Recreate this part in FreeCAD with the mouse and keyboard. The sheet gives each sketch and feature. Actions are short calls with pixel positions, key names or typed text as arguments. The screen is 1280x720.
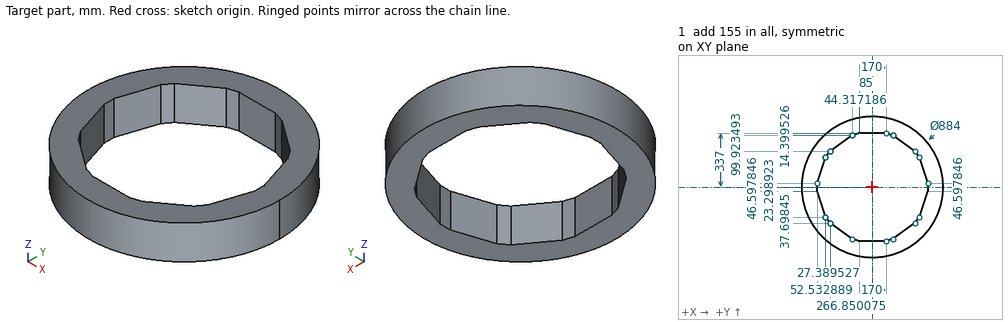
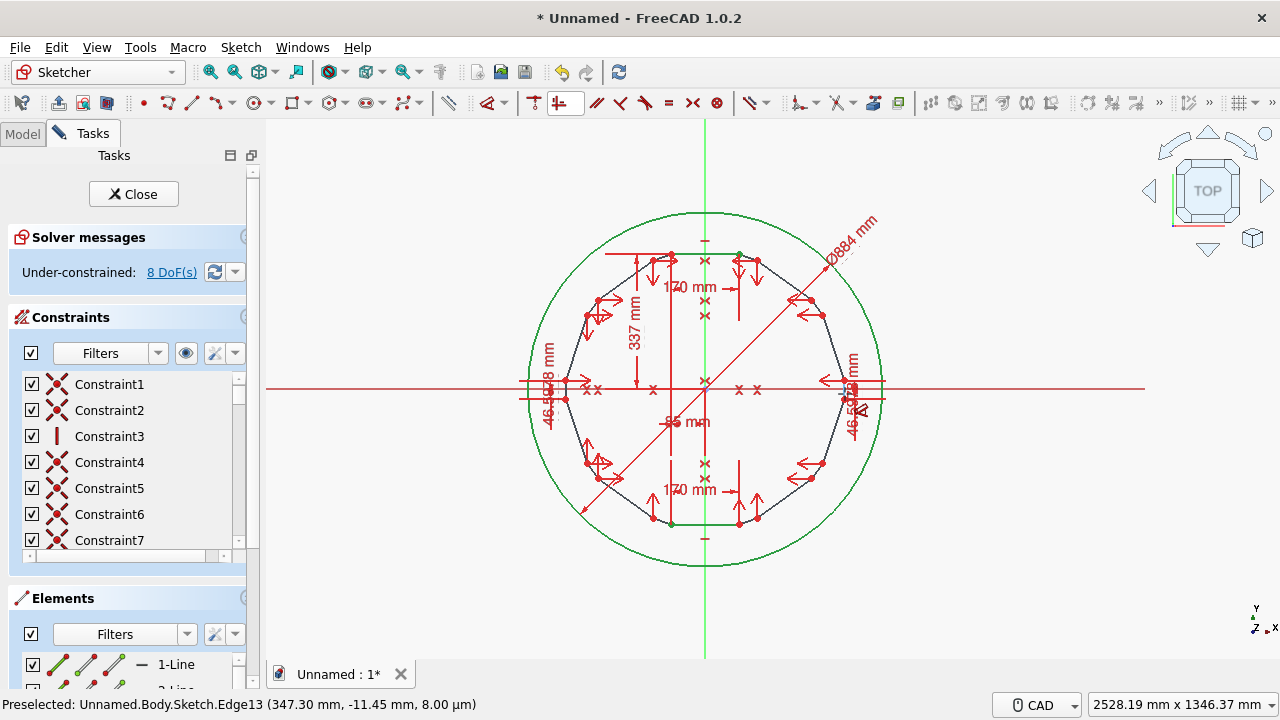
scroll(595, 474, up, 5)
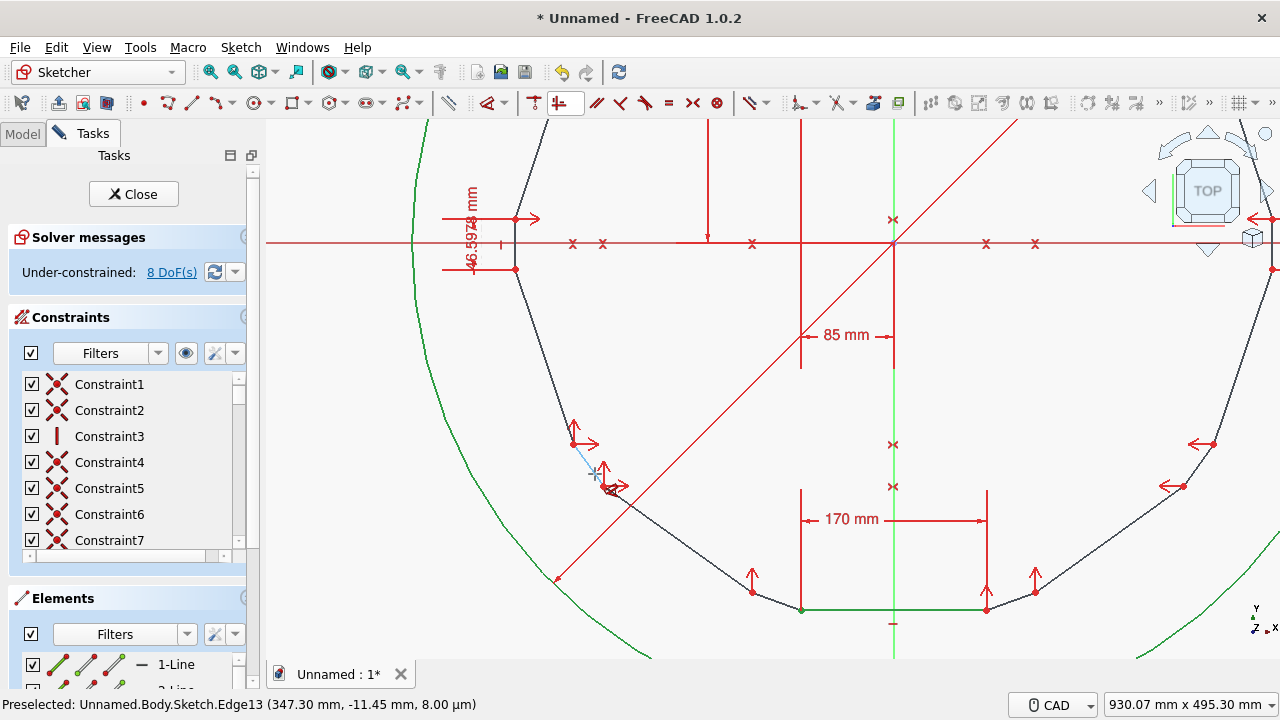
click(595, 474)
click(540, 465)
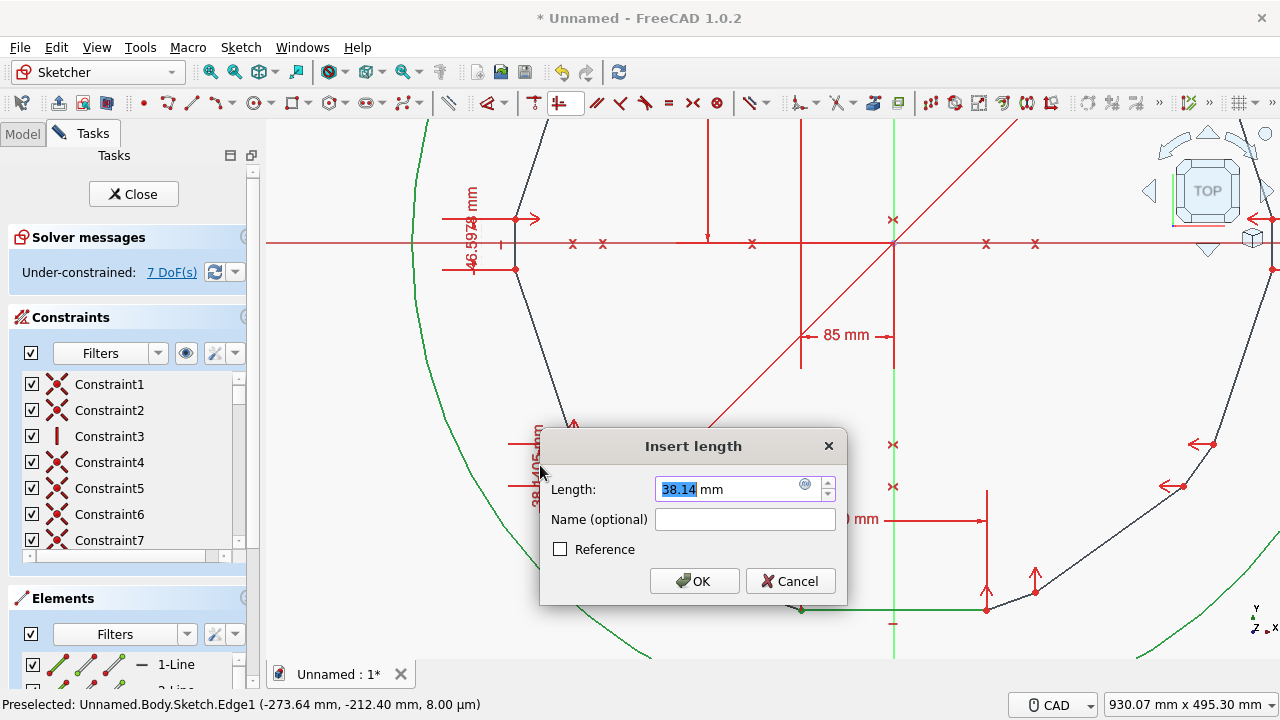
text(37.69845)
key(Return)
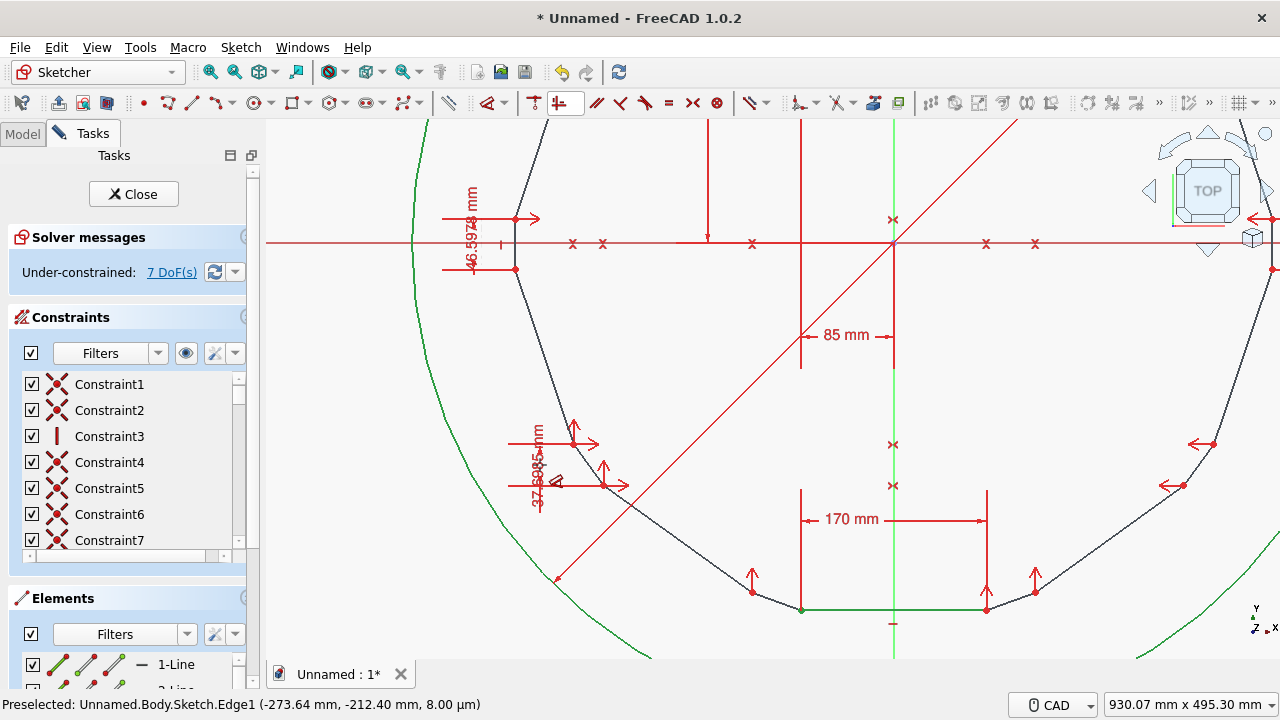
scroll(515, 270, up, 3)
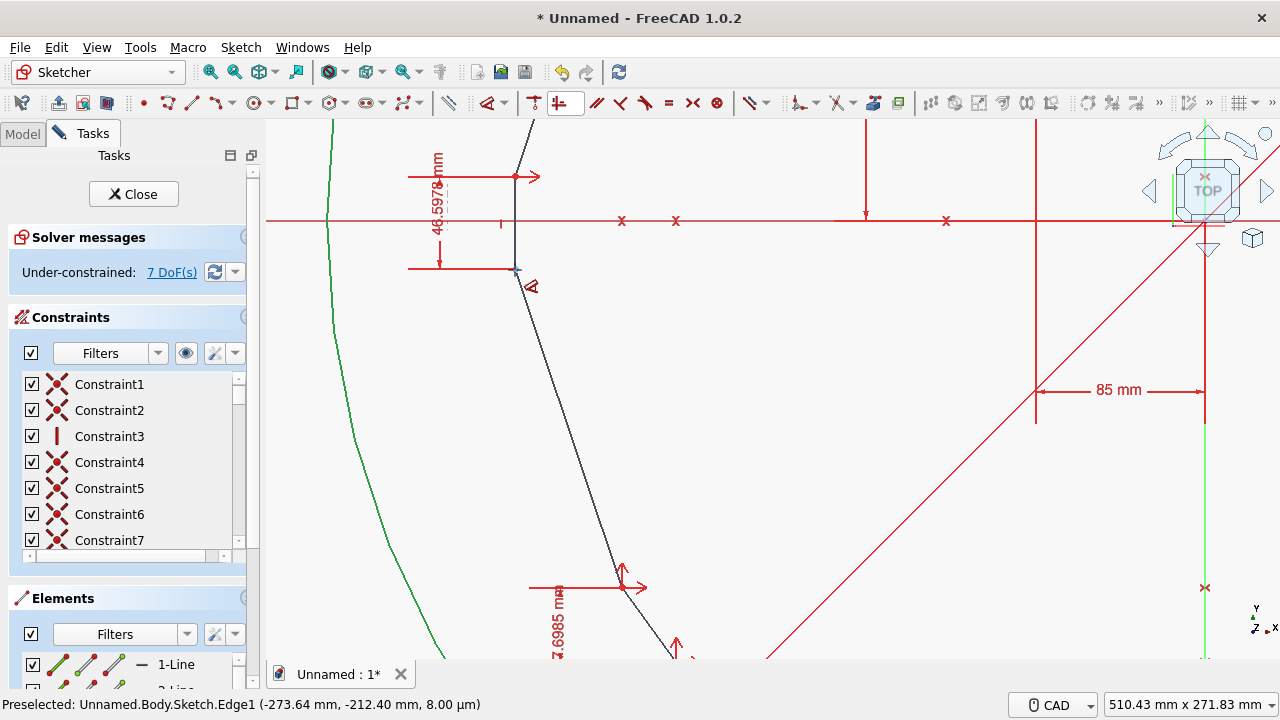
click(515, 269)
click(481, 245)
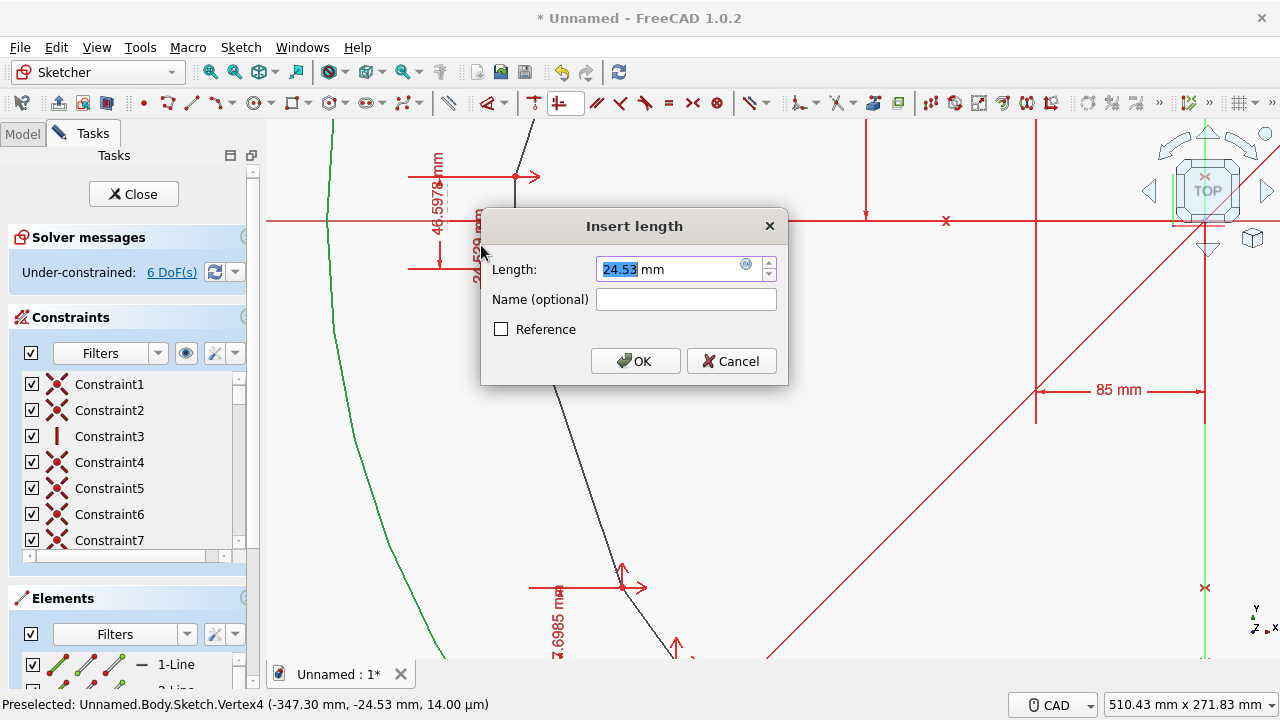
text(23.298923)
key(Return)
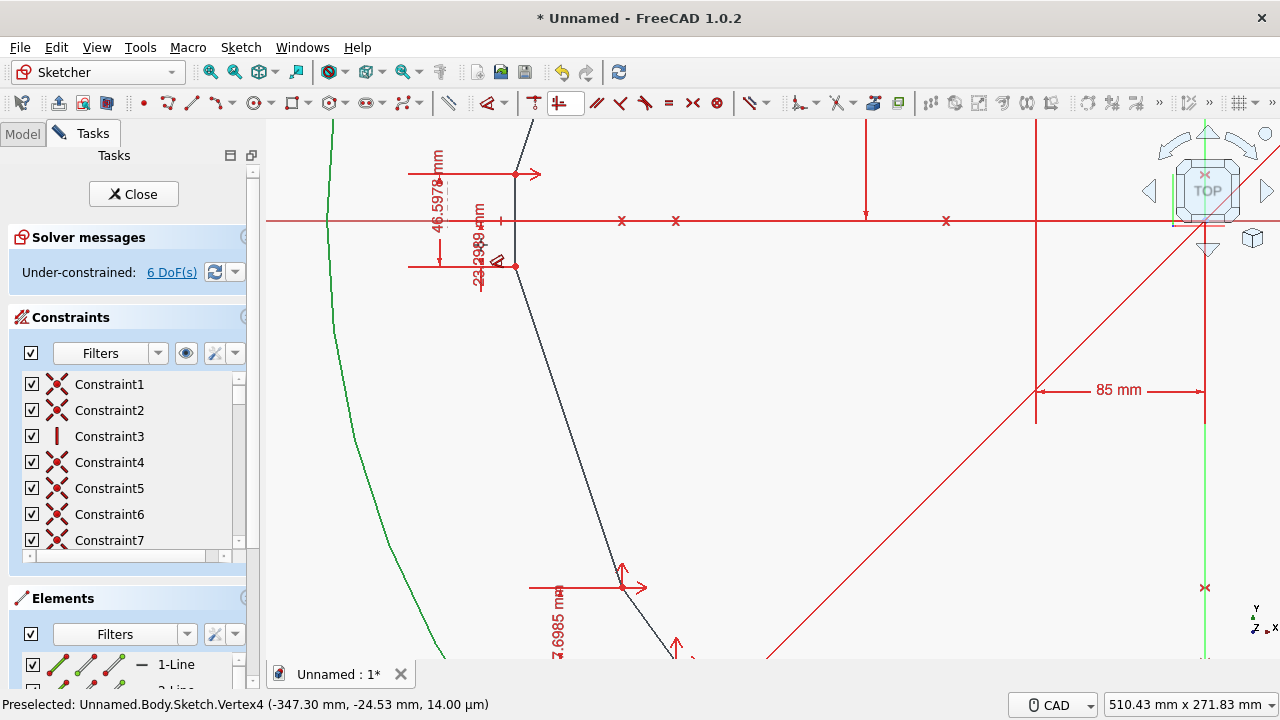
click(638, 610)
click(649, 554)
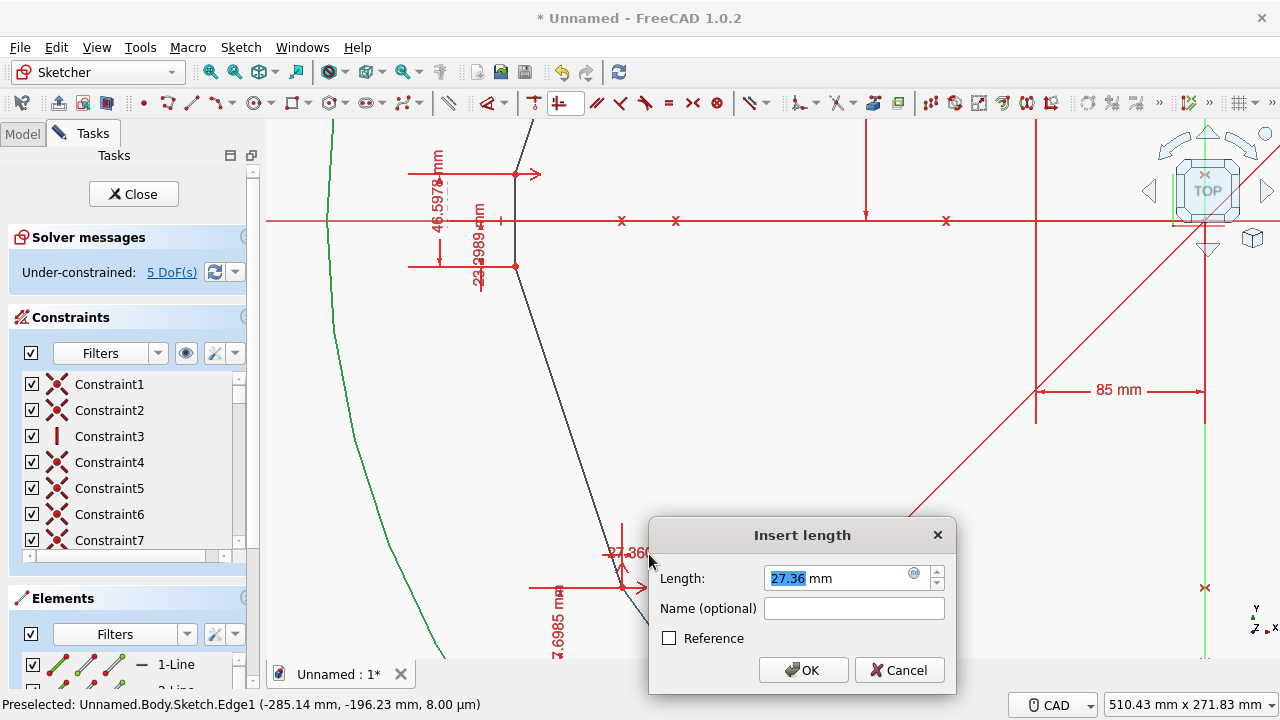
text(27.389527)
key(Return)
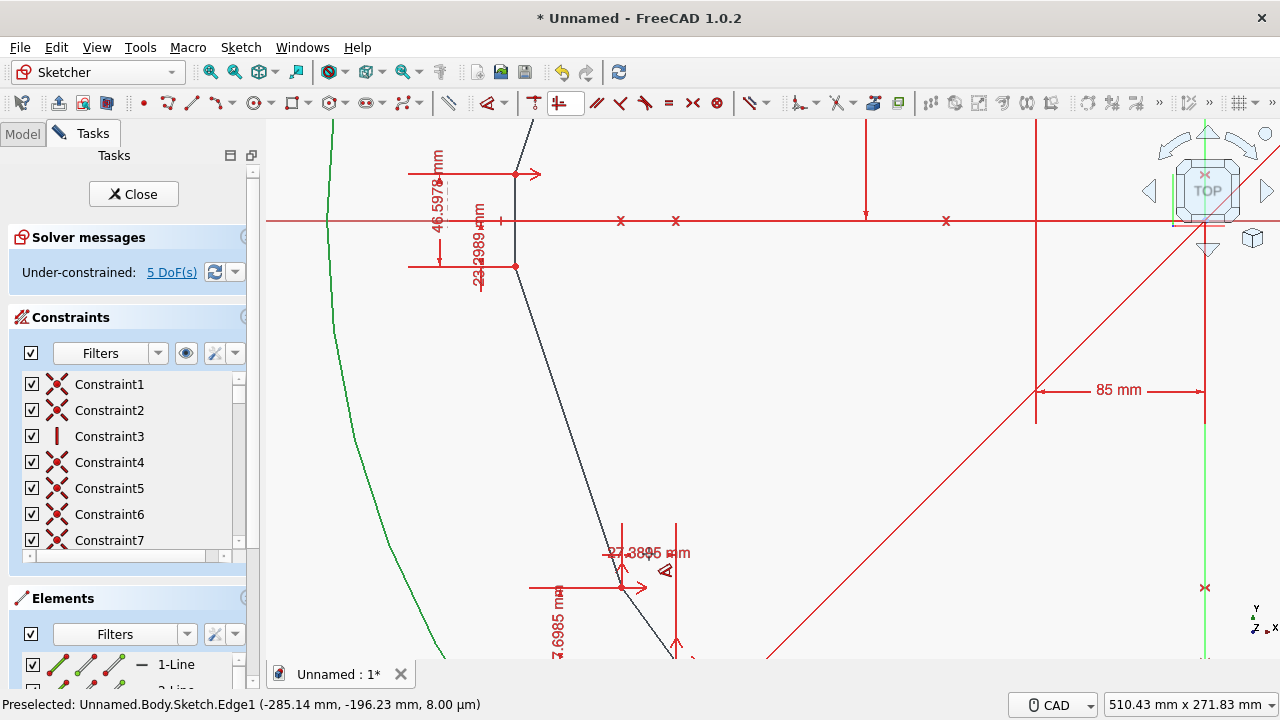
click(590, 491)
click(569, 185)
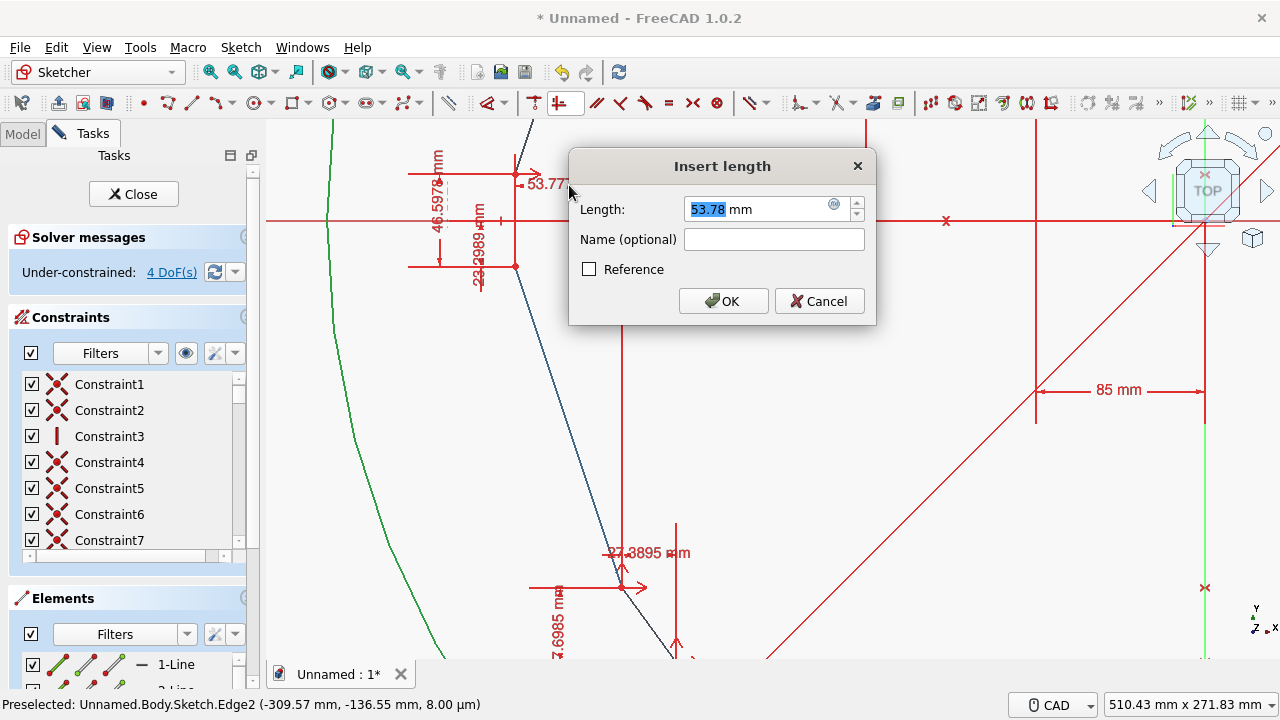
text(52.532889)
key(Return)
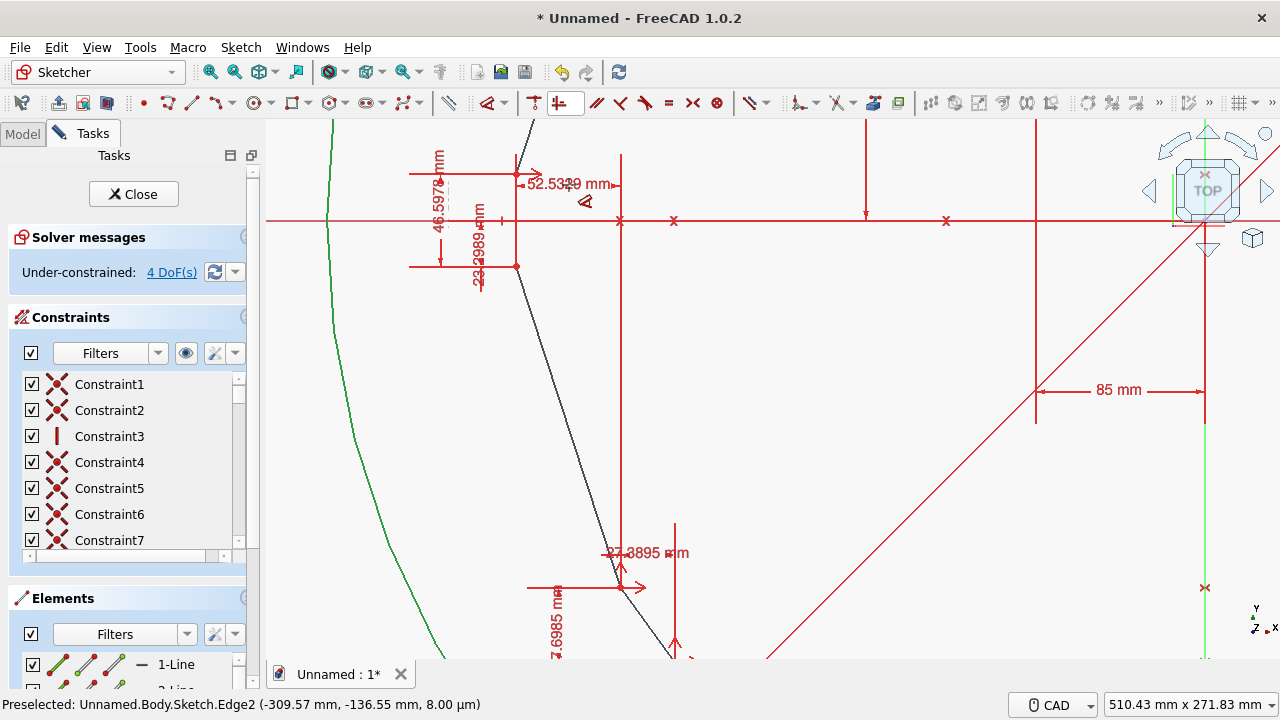
scroll(578, 432, down, 8)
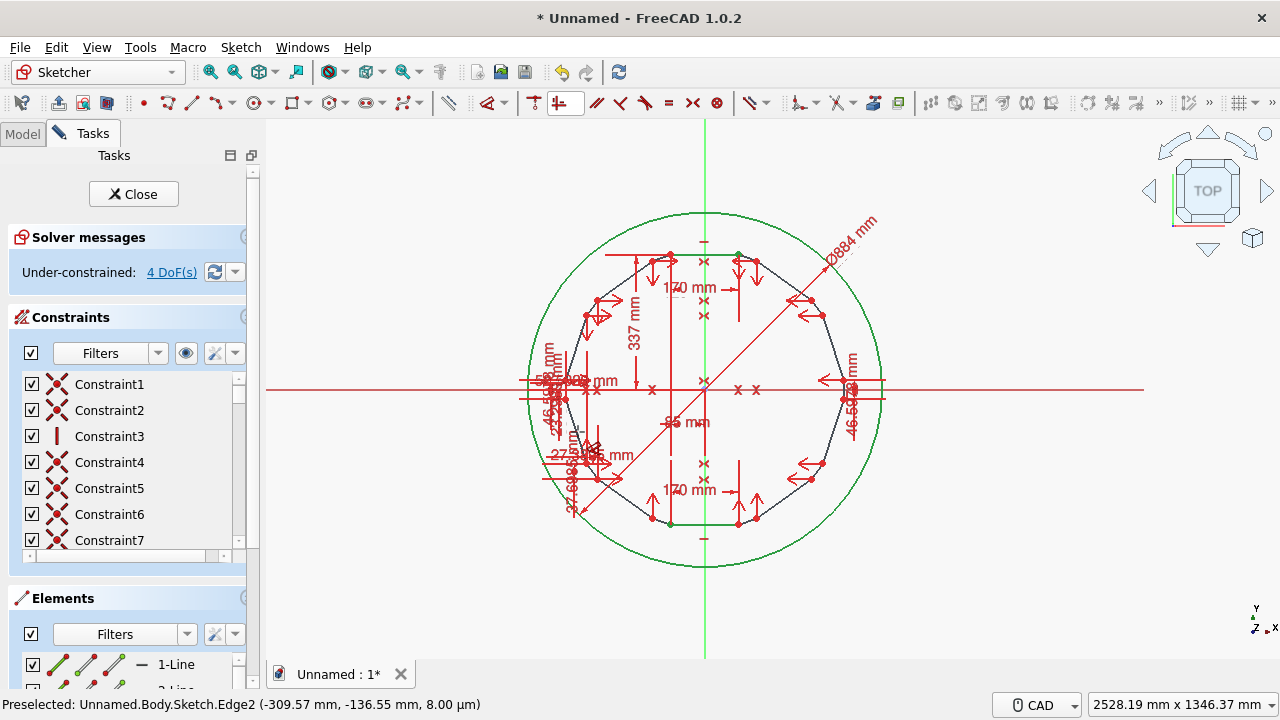
click(614, 289)
click(540, 281)